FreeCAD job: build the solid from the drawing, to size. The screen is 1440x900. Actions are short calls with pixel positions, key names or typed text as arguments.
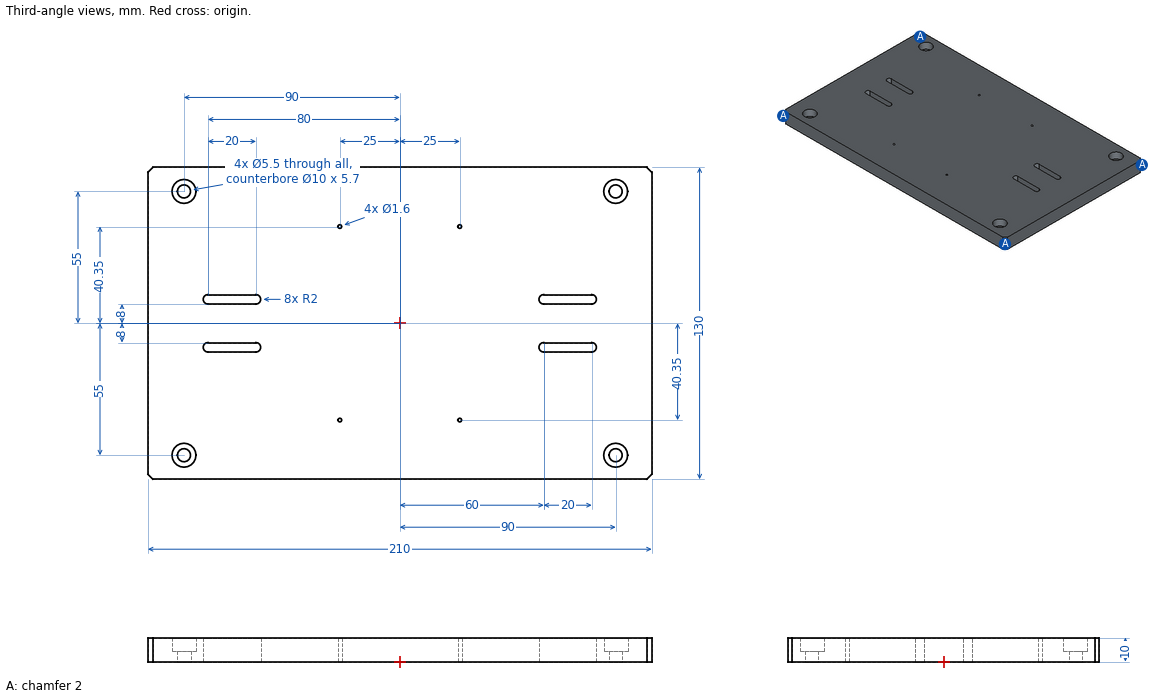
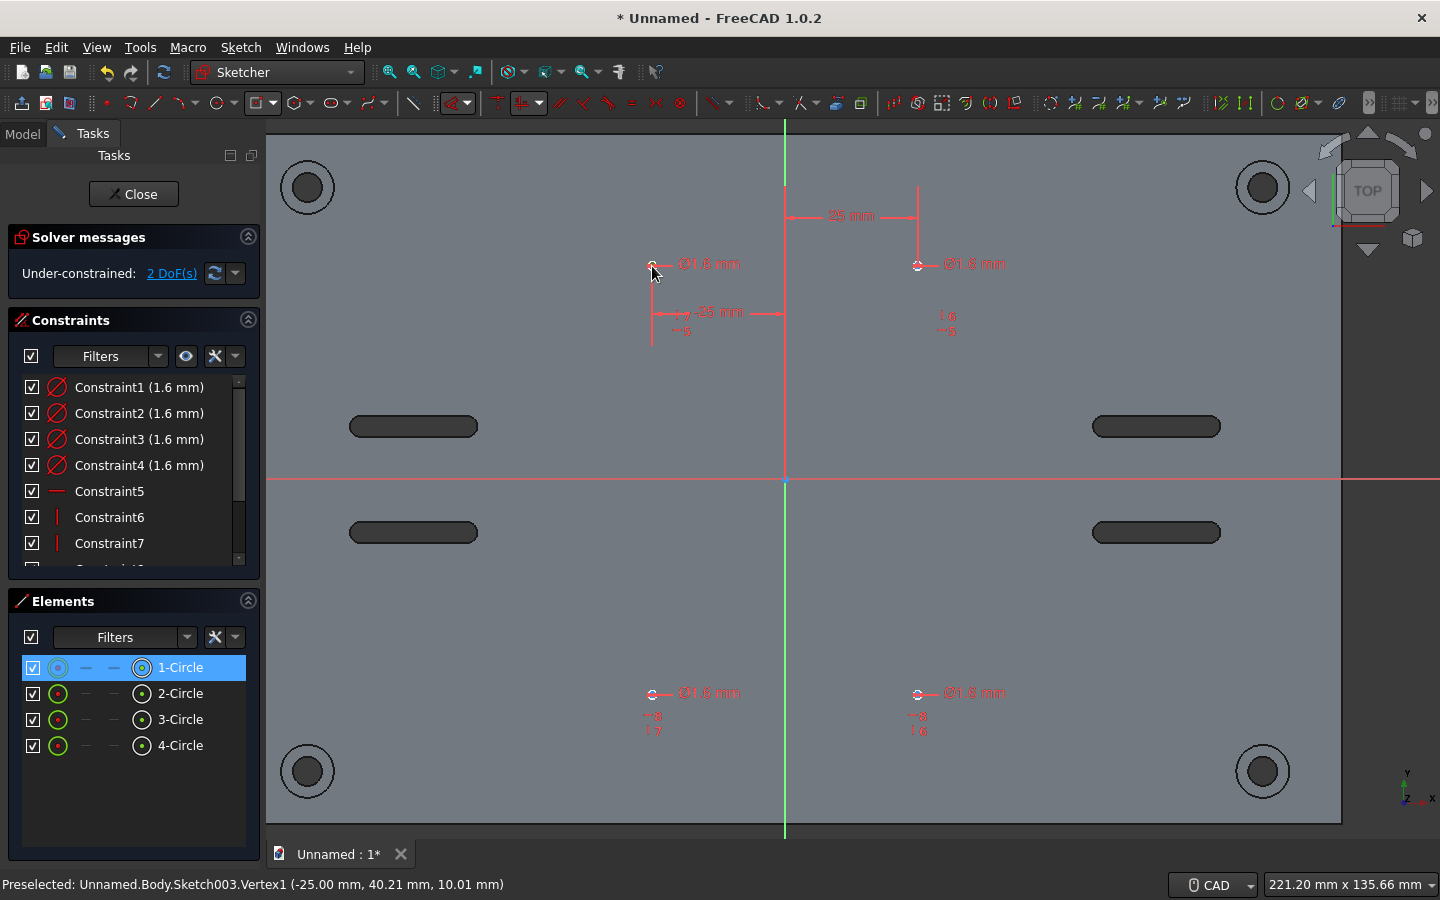
click(470, 104)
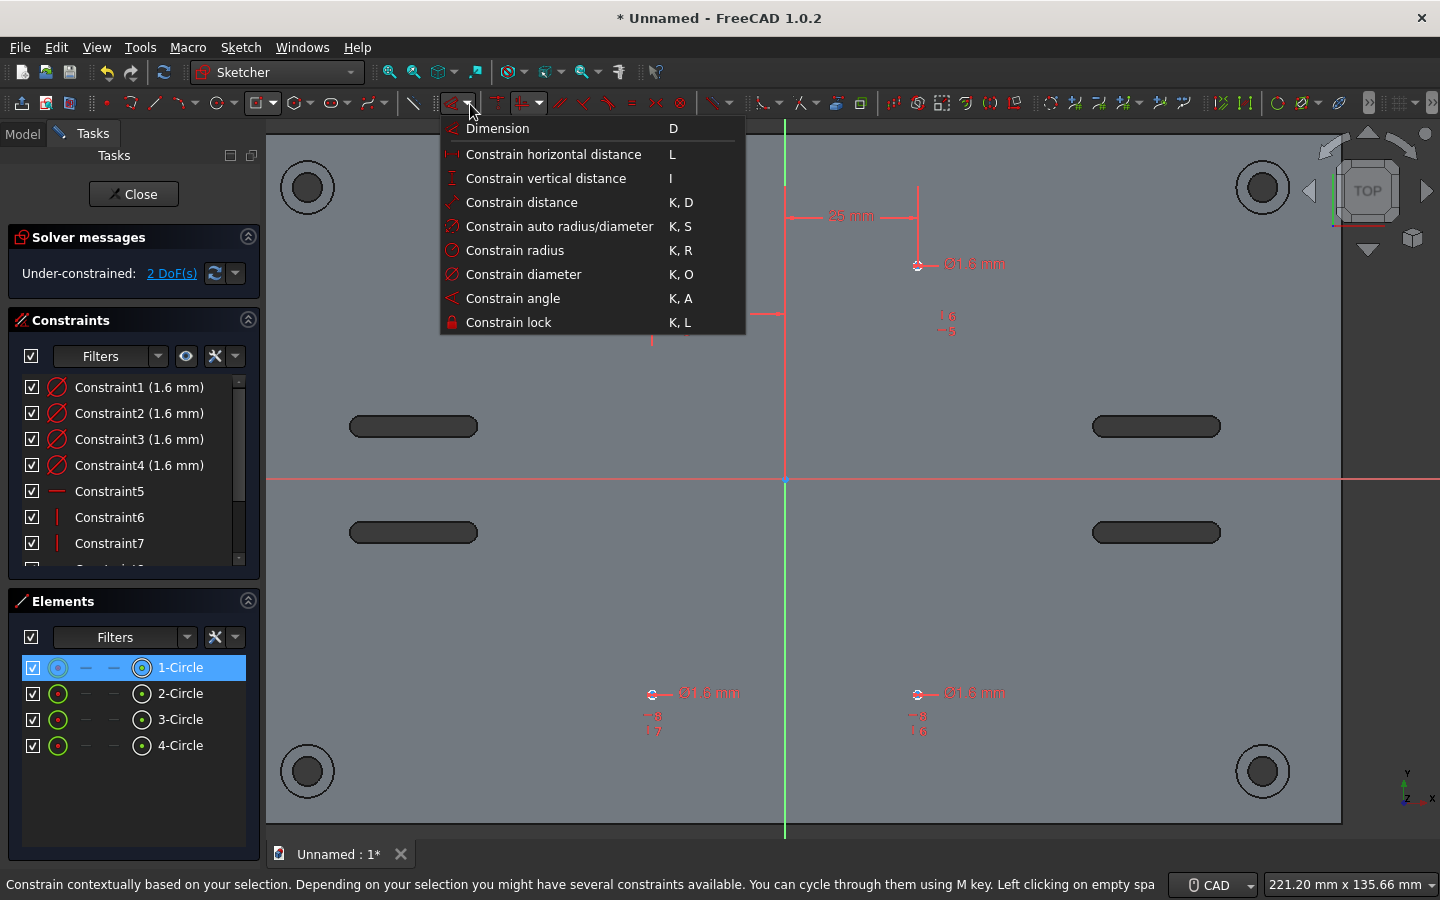
click(593, 178)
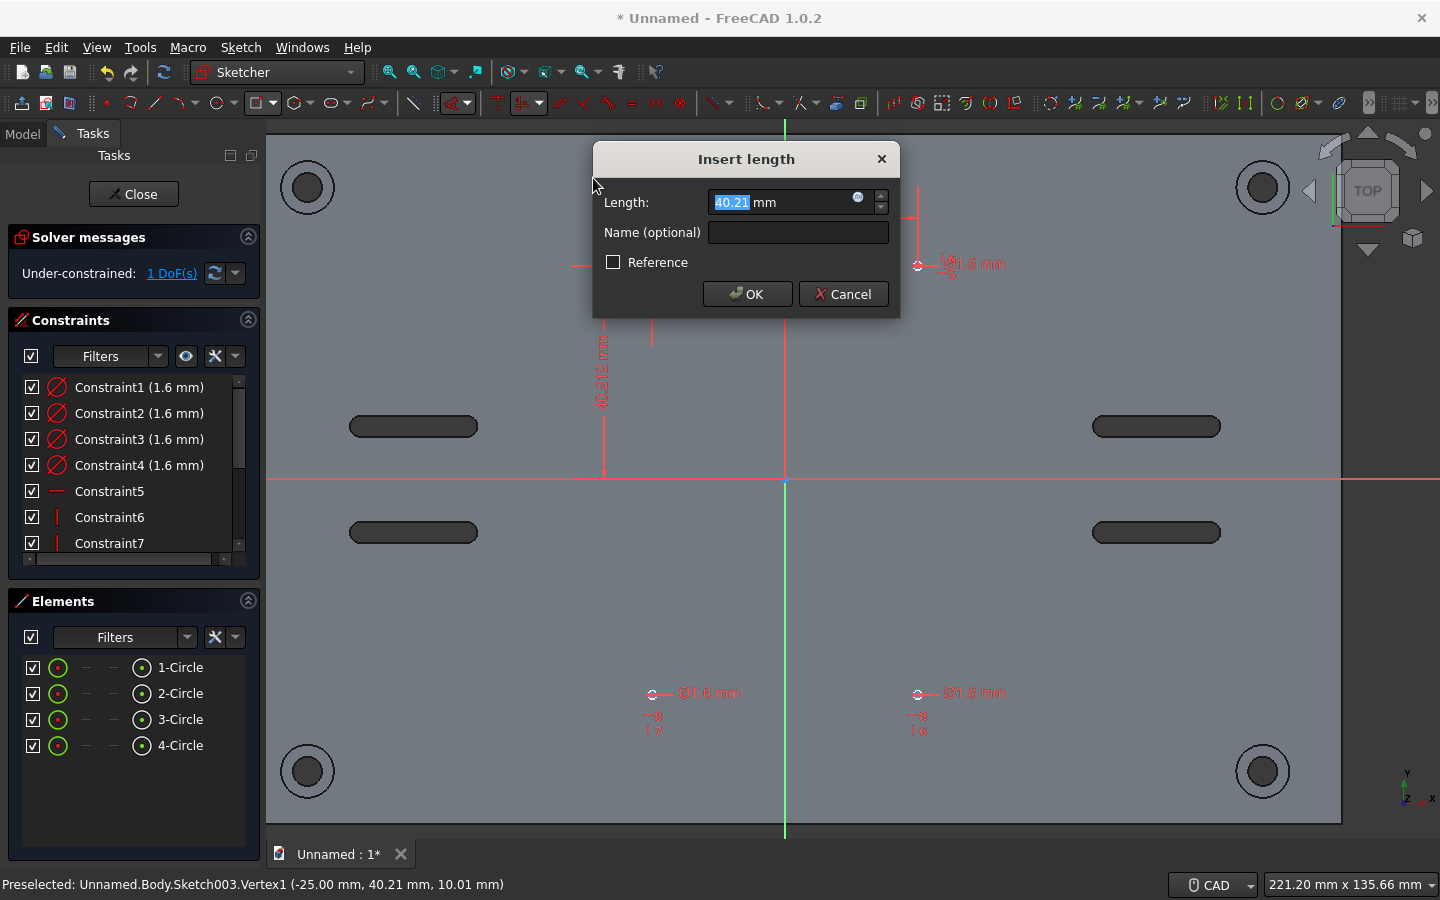
text(40.35)
key(Return)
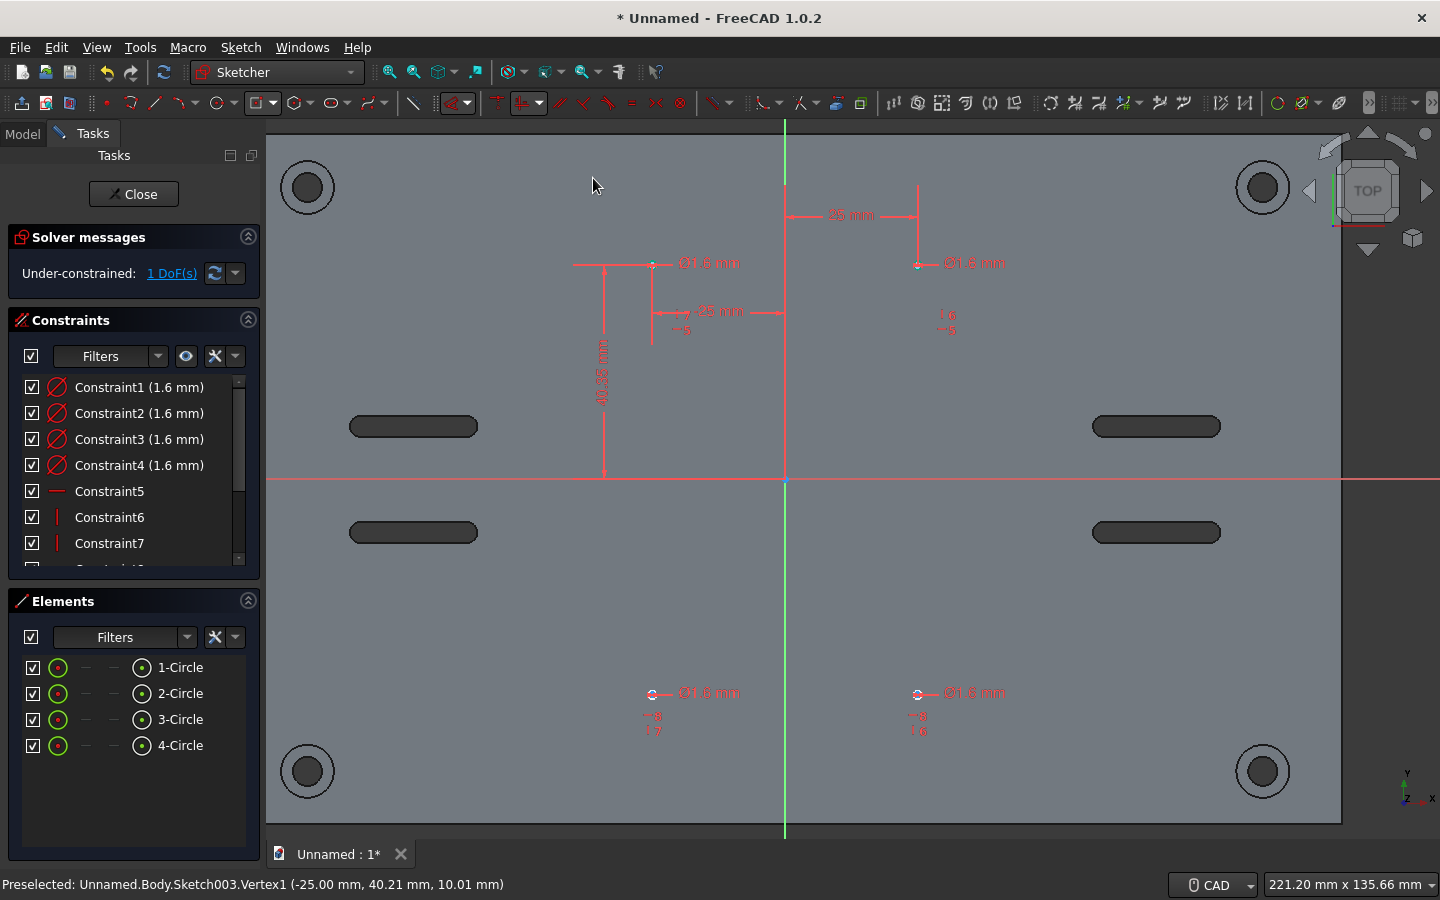
click(918, 695)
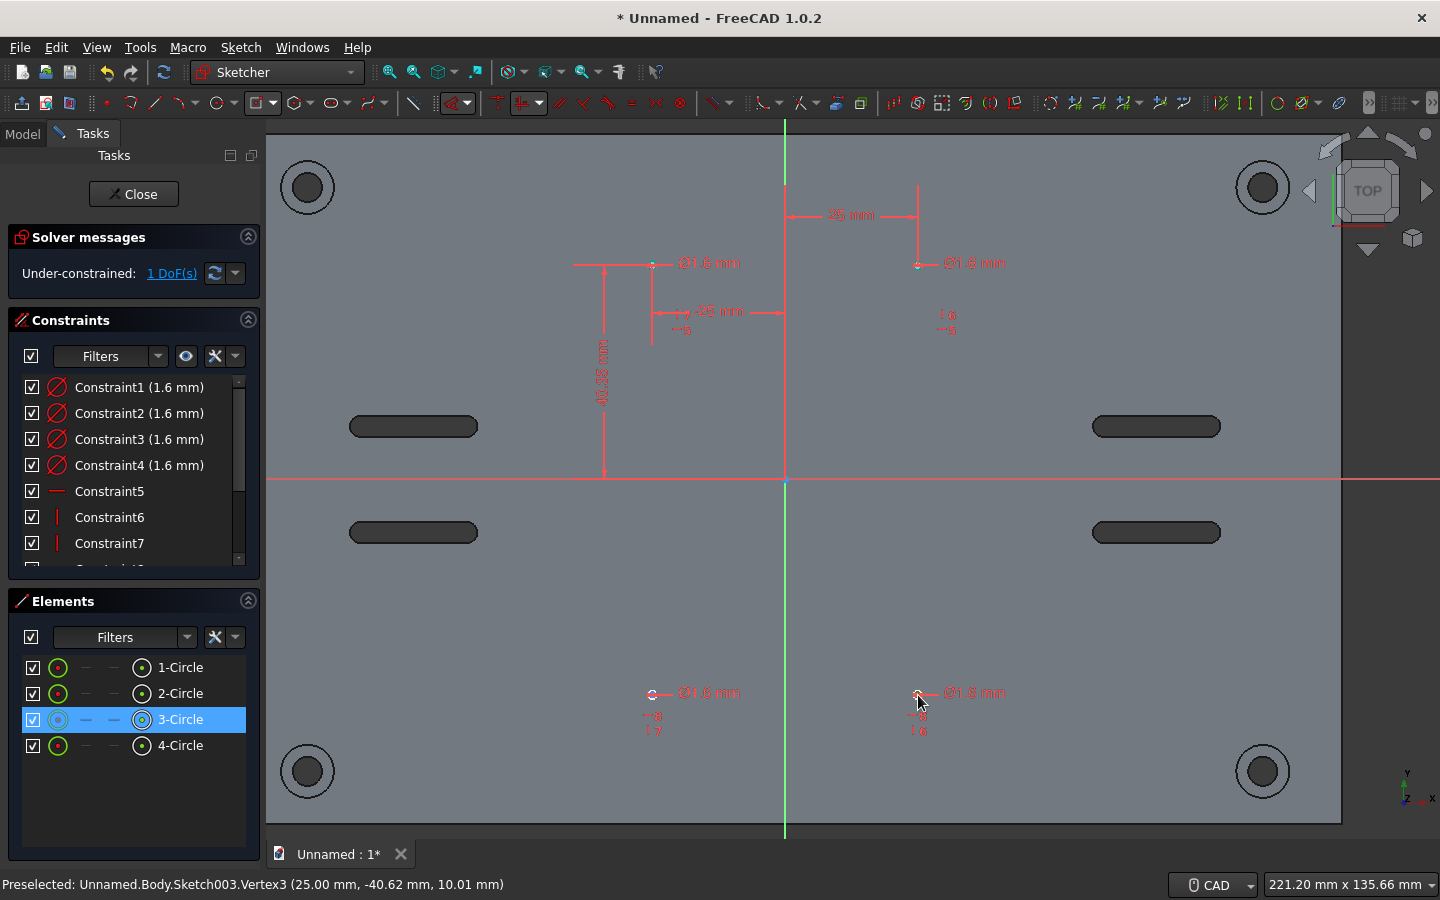
key(i)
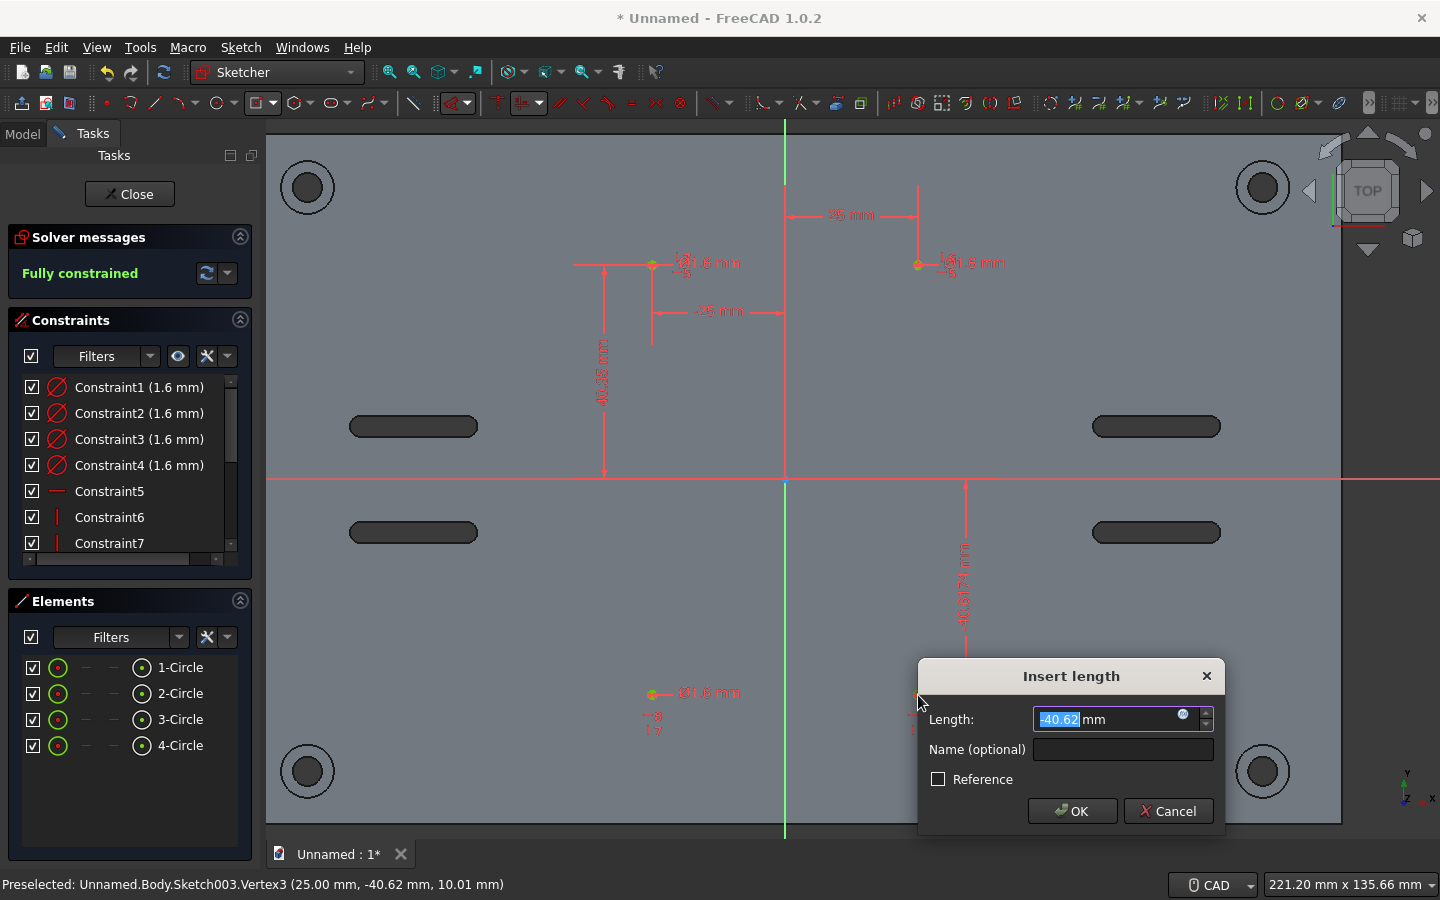
text(-40.35)
key(Return)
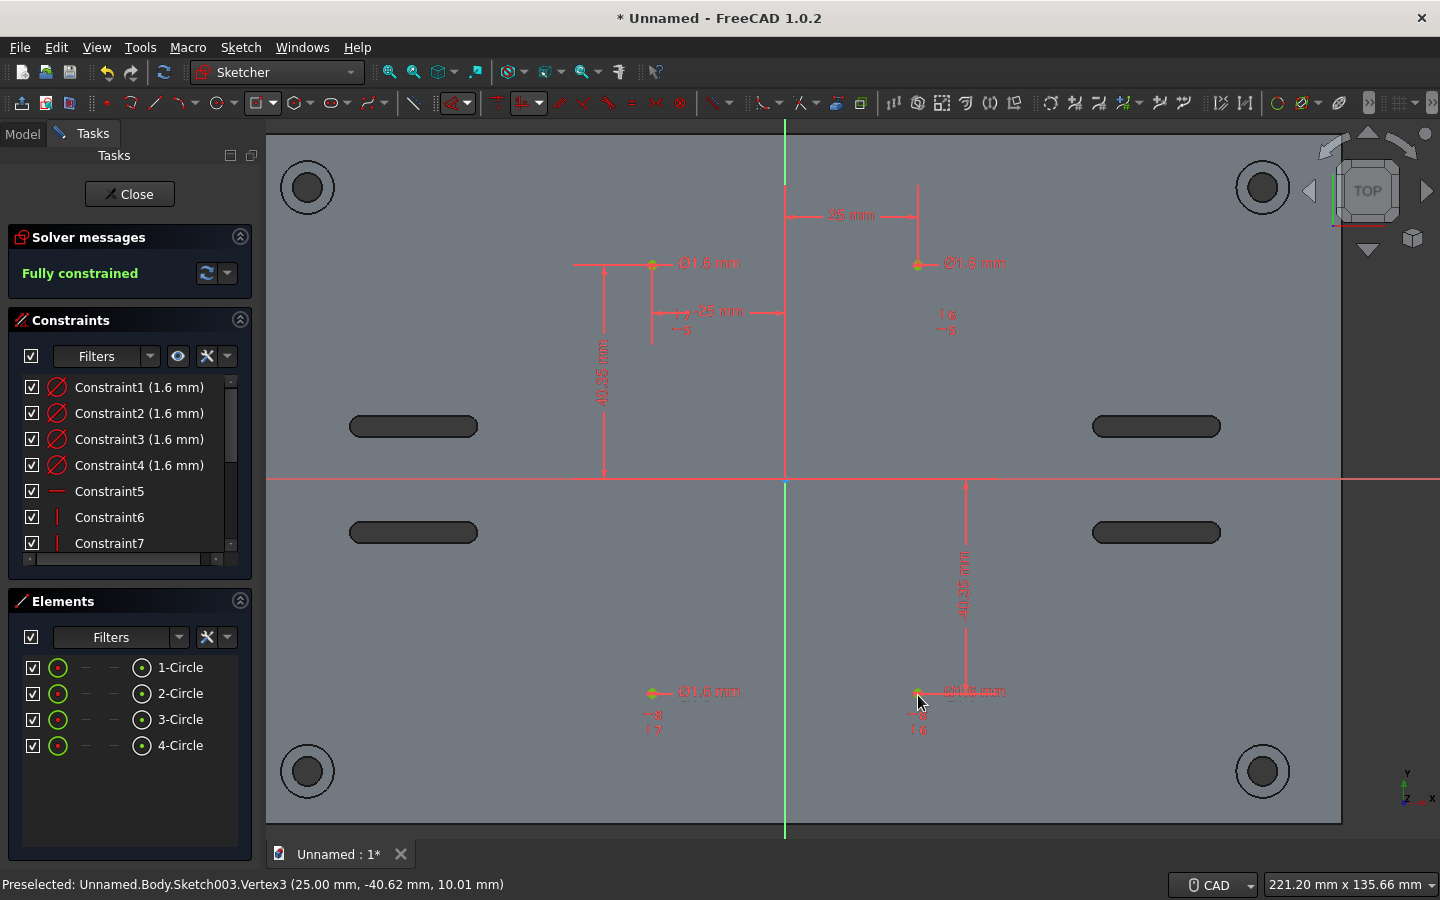
click(130, 194)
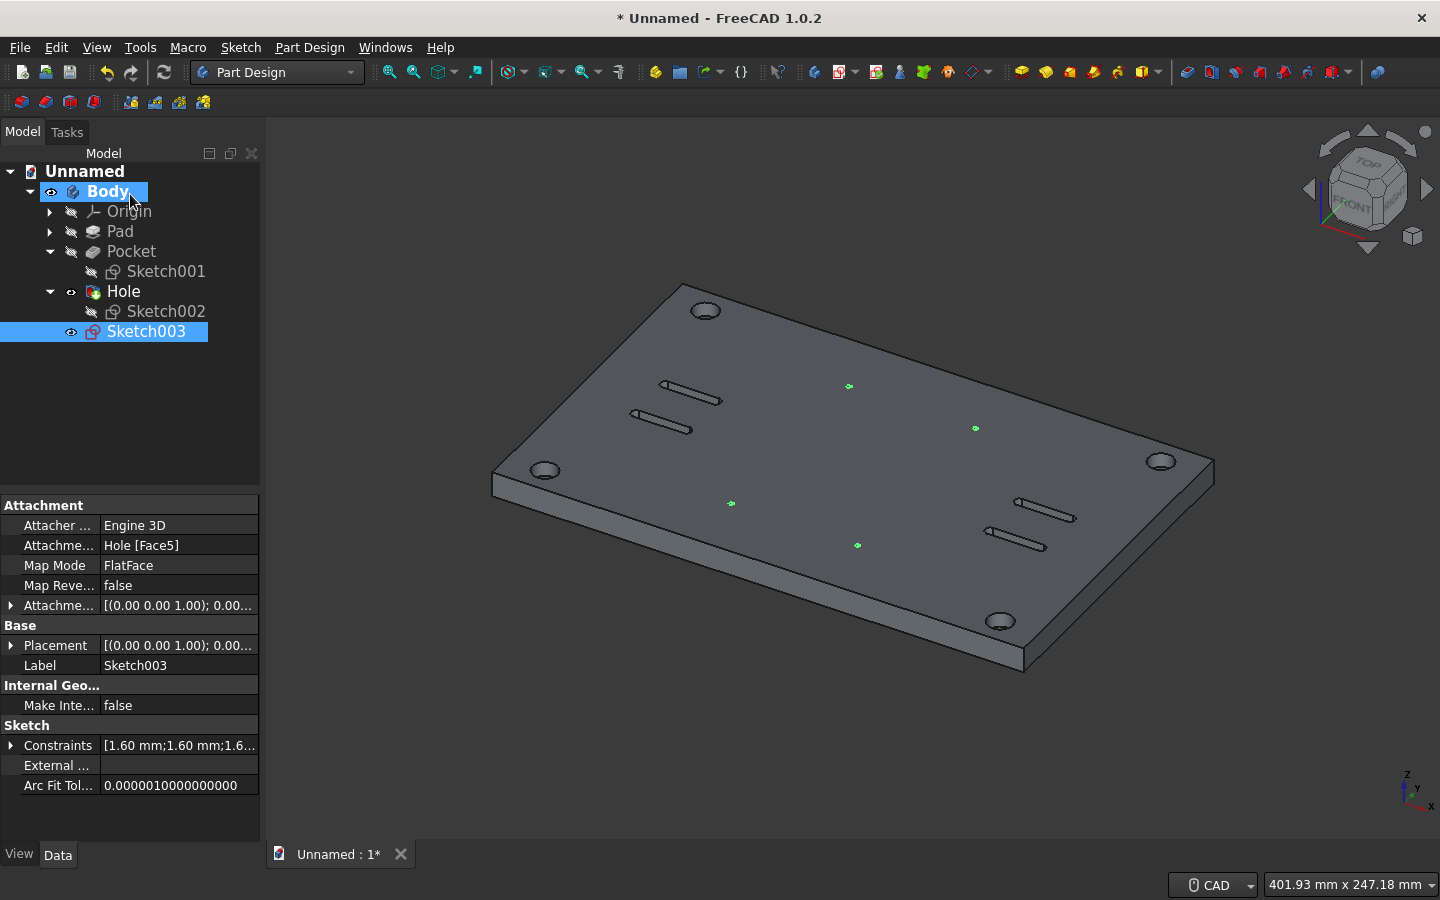
click(1188, 72)